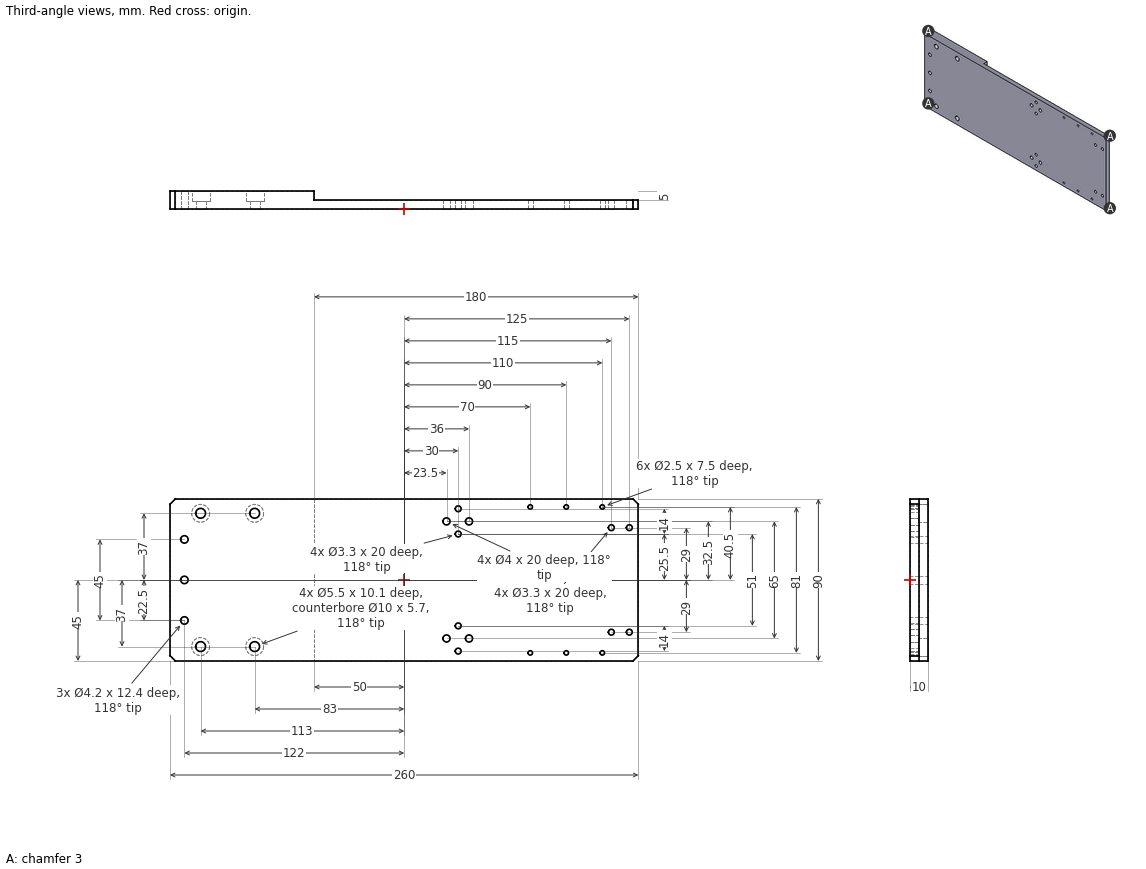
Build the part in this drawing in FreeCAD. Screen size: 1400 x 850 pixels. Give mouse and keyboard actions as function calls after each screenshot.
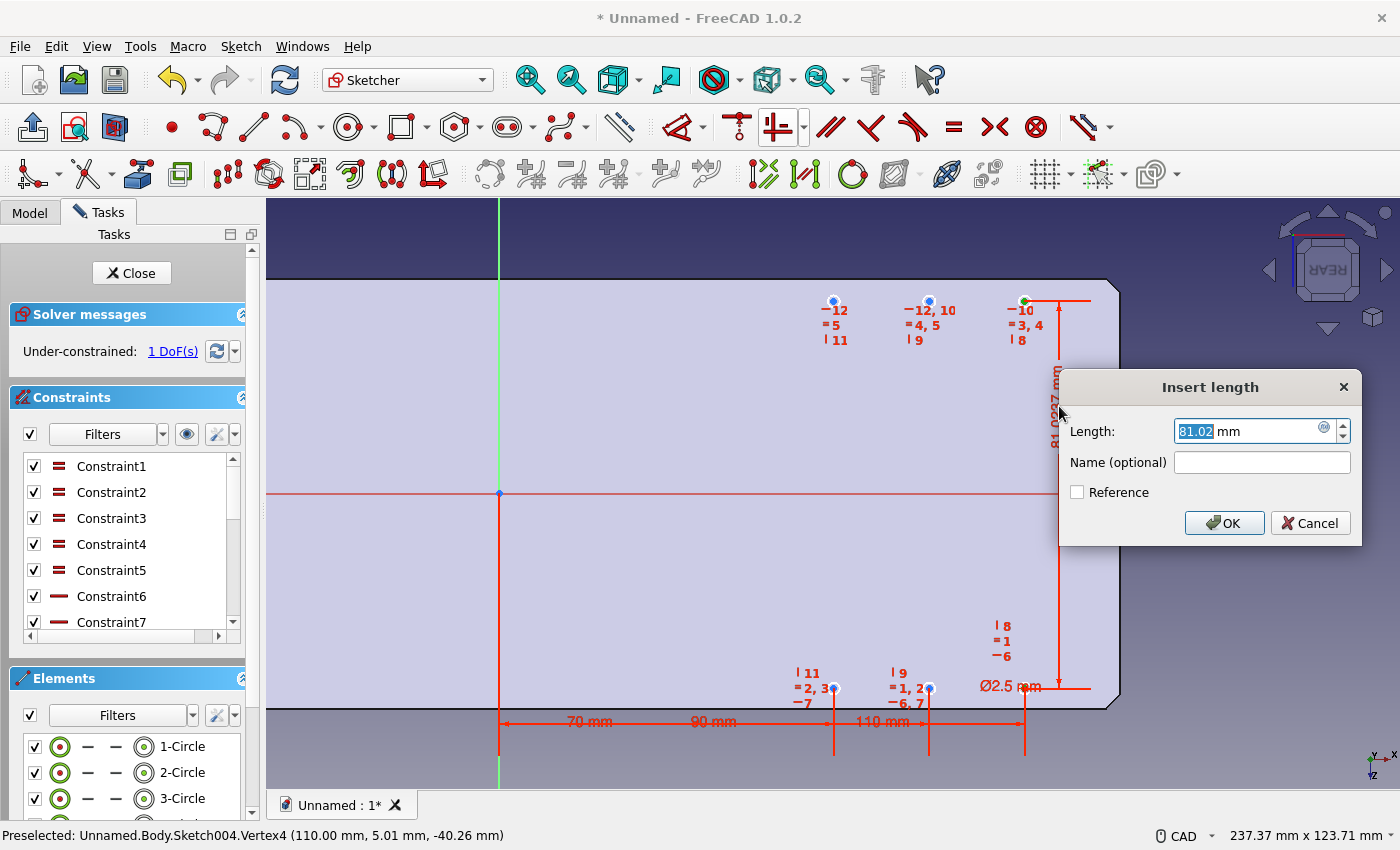
text(81)
key(Return)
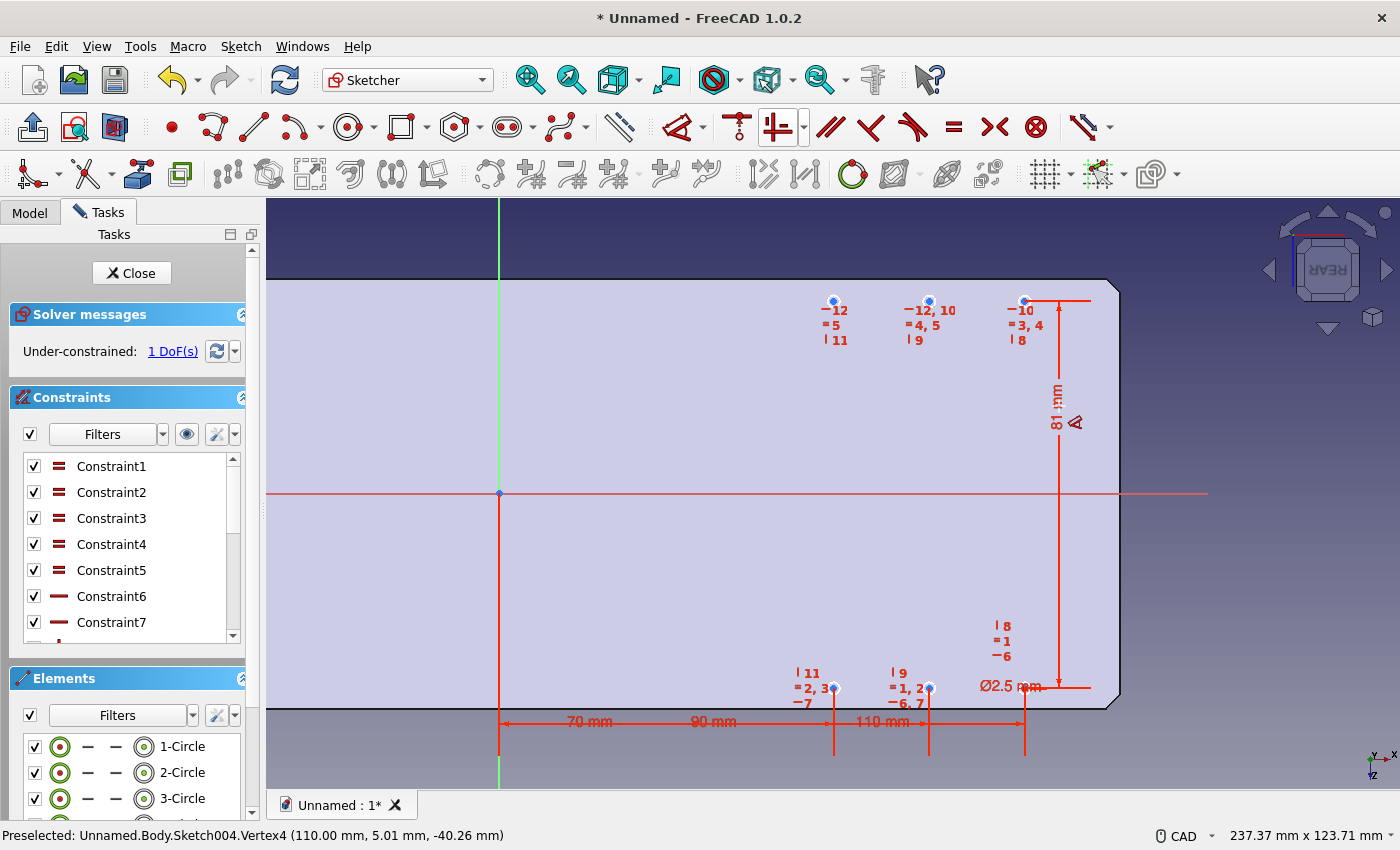
click(1025, 688)
click(465, 591)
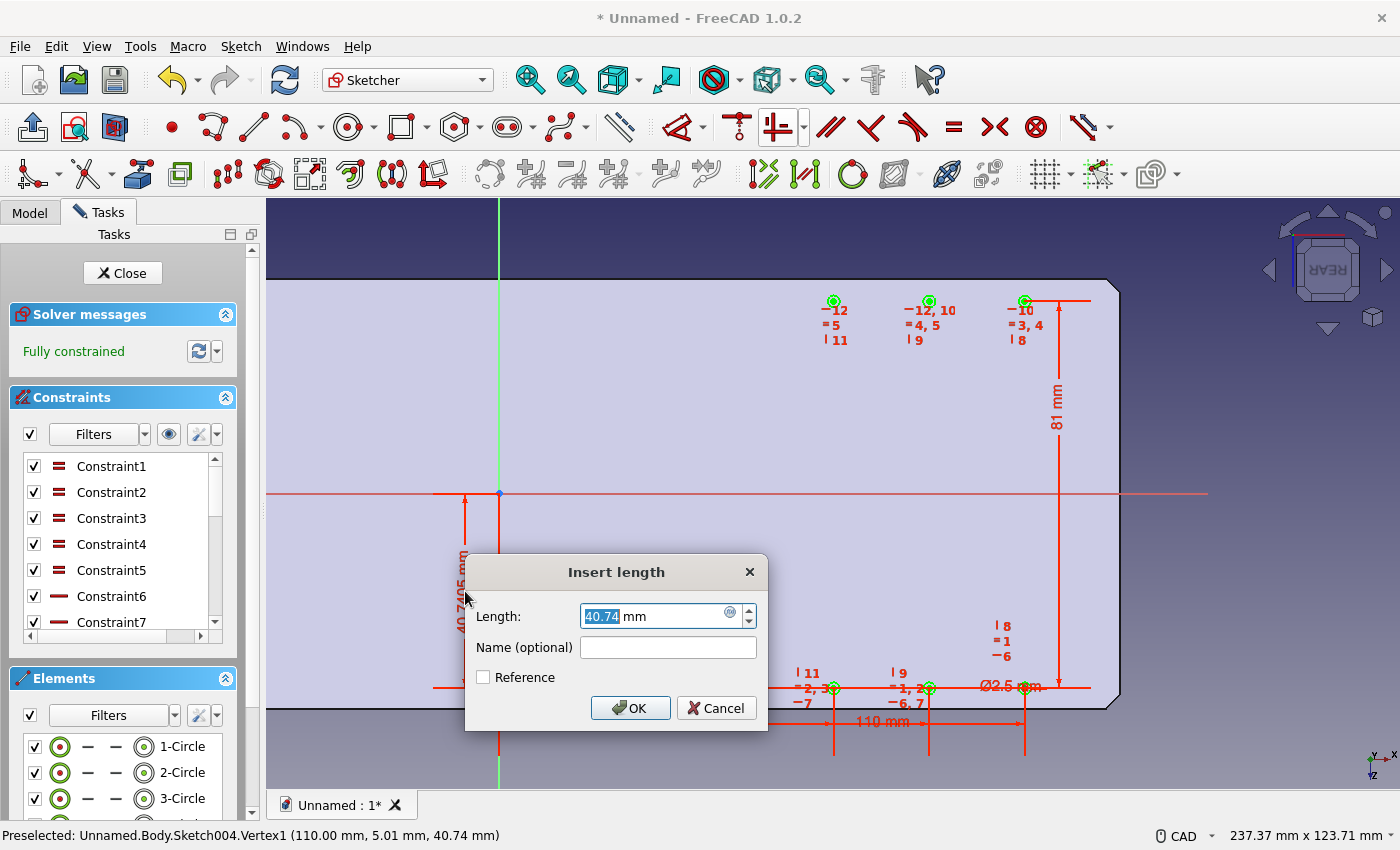
text(40.5)
key(Return)
key(Escape)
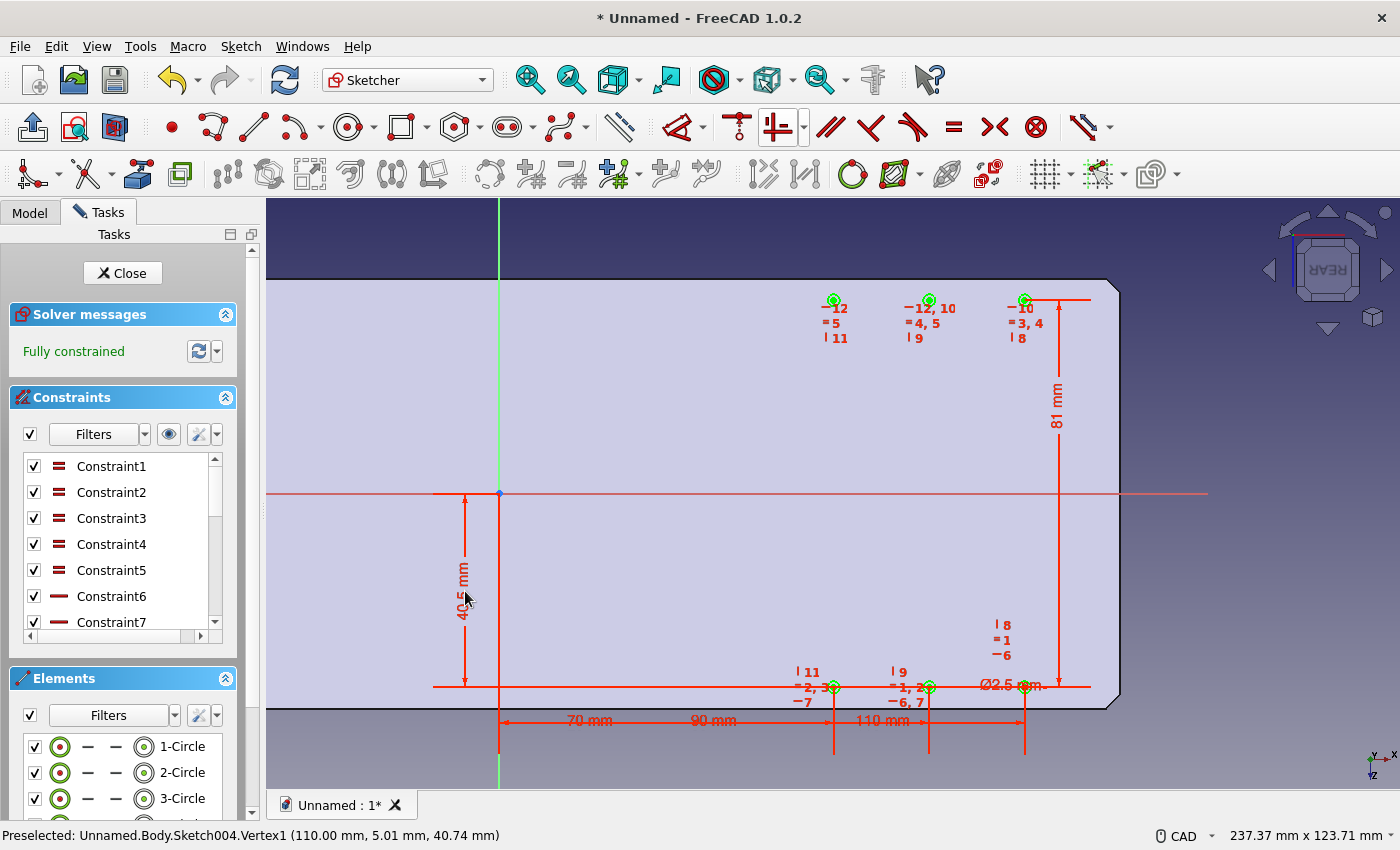
click(123, 273)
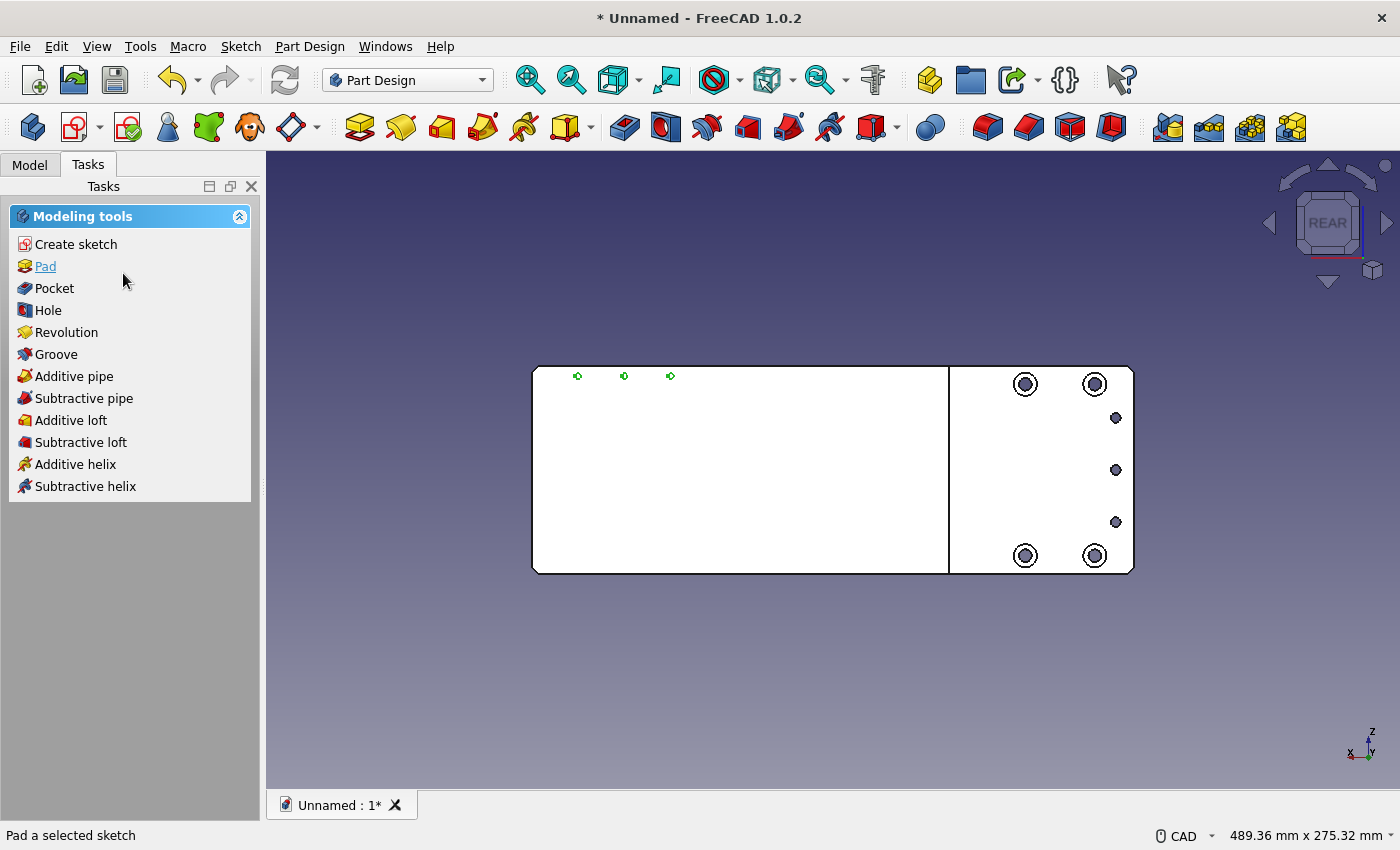
click(666, 128)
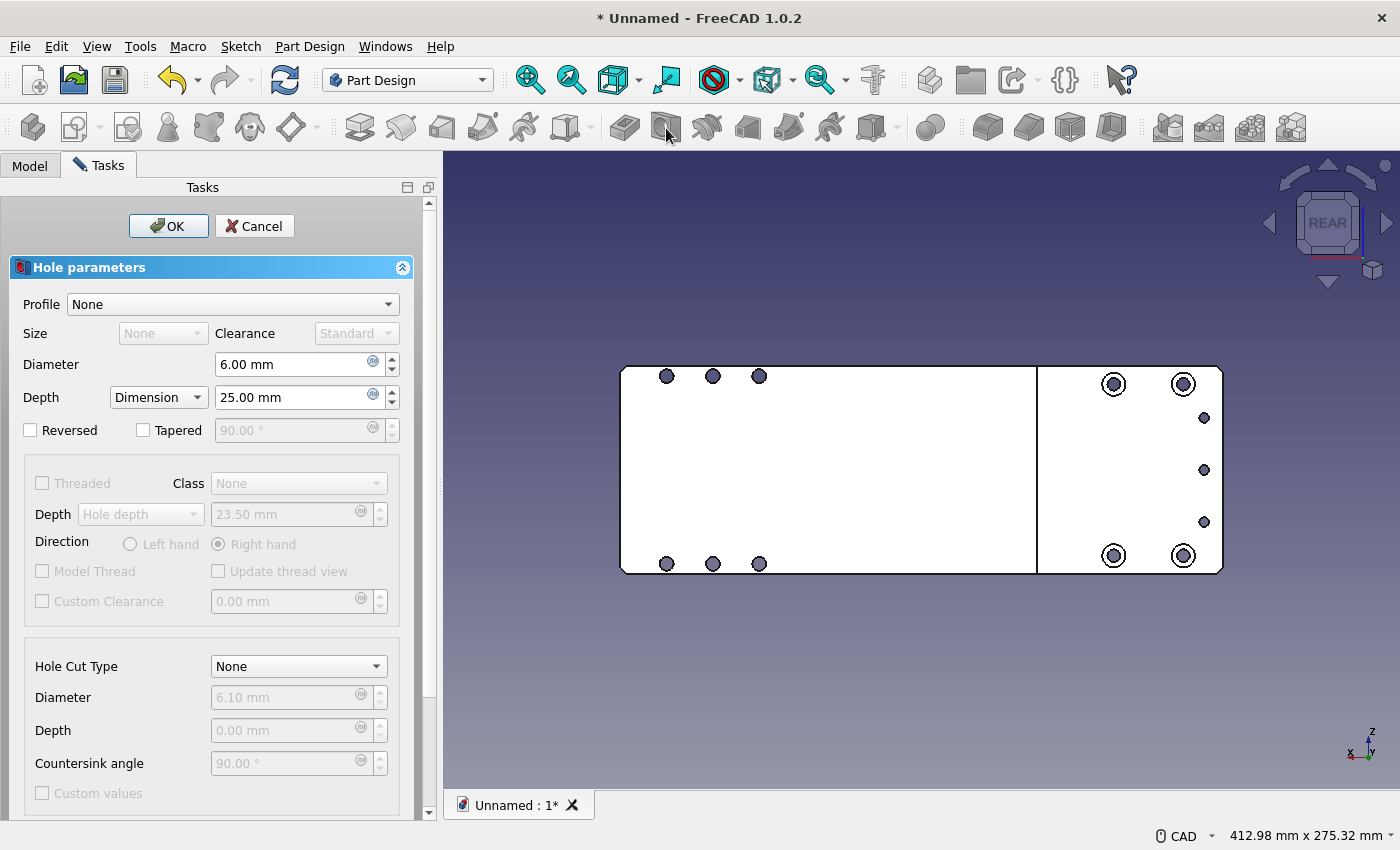
triple_click(300, 364)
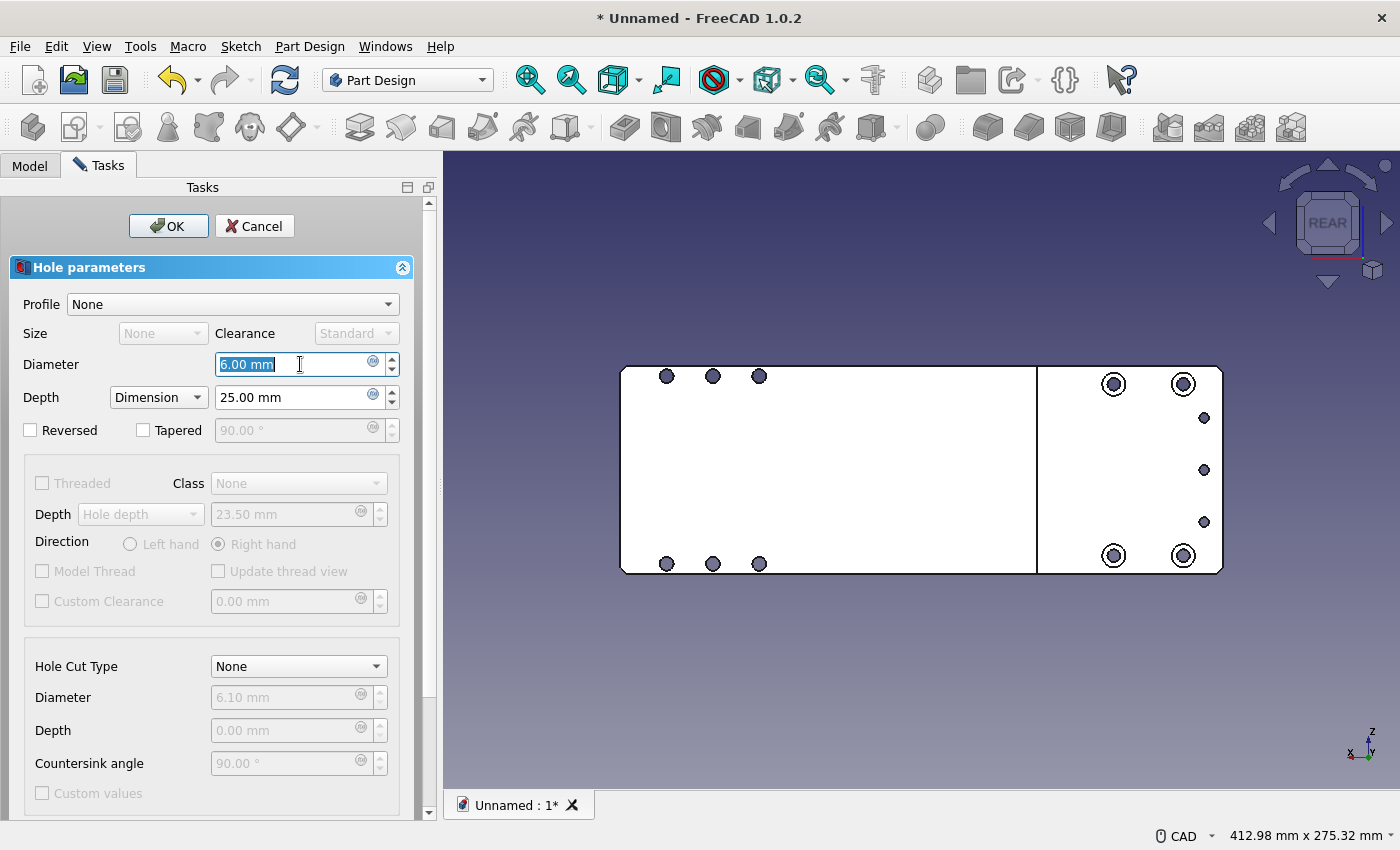
text(2.5)
key(Tab)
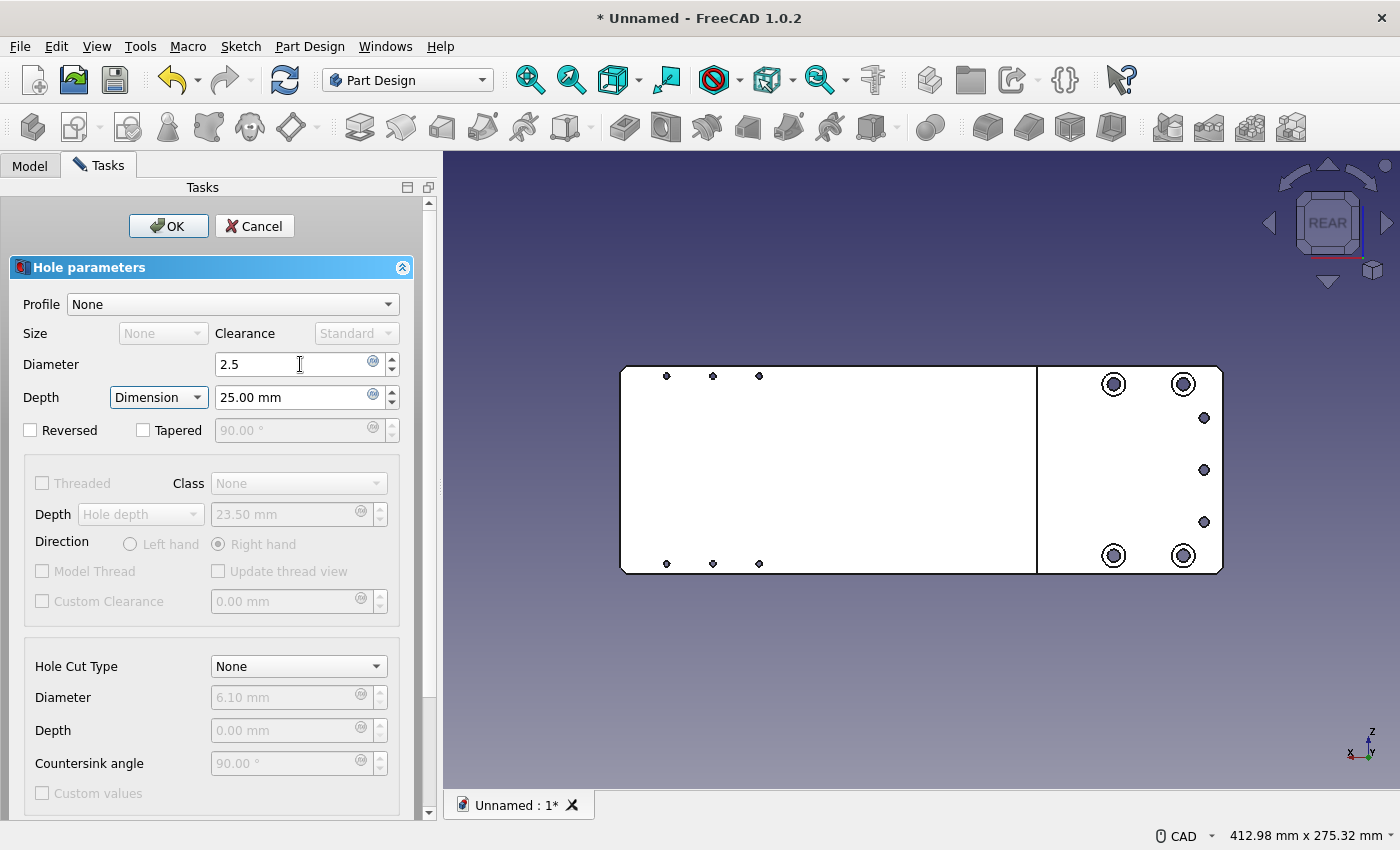
triple_click(300, 398)